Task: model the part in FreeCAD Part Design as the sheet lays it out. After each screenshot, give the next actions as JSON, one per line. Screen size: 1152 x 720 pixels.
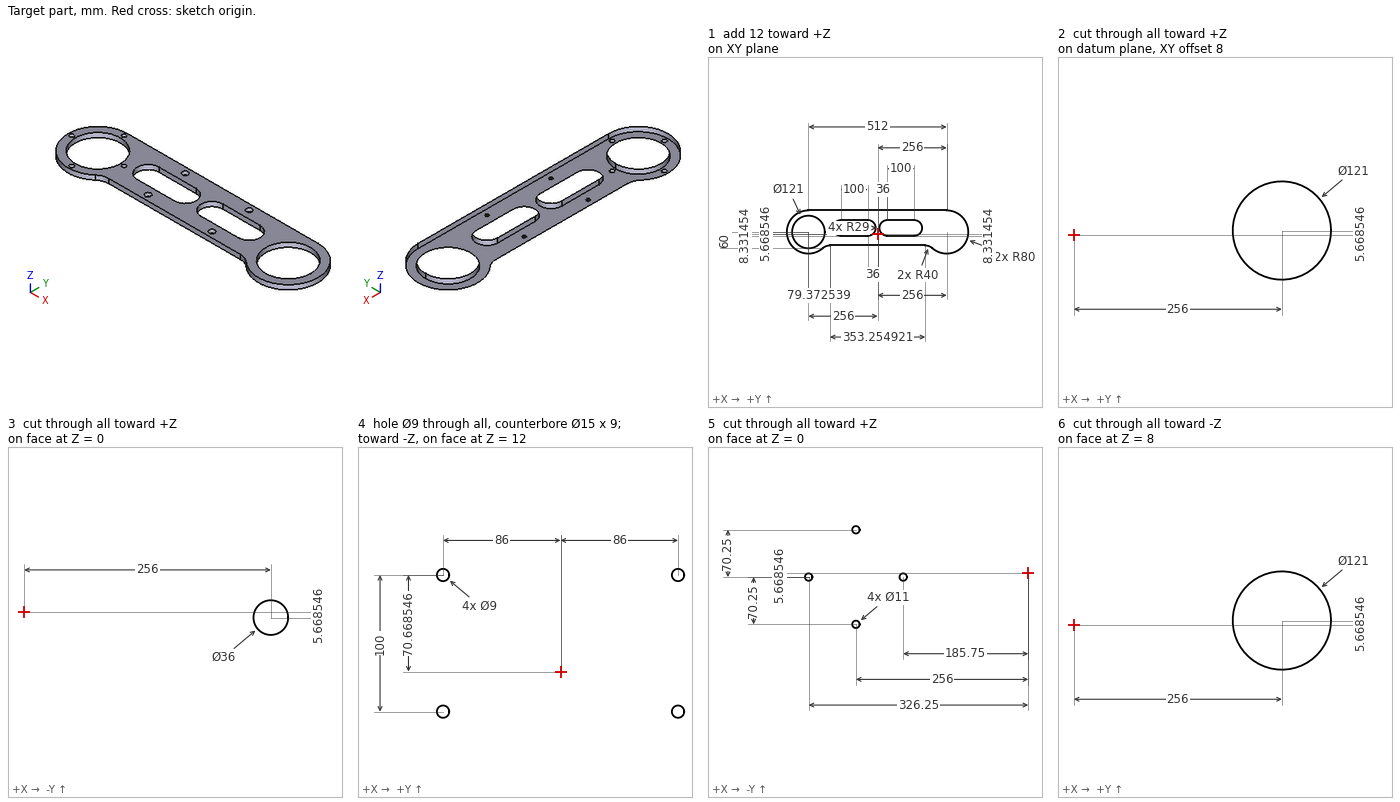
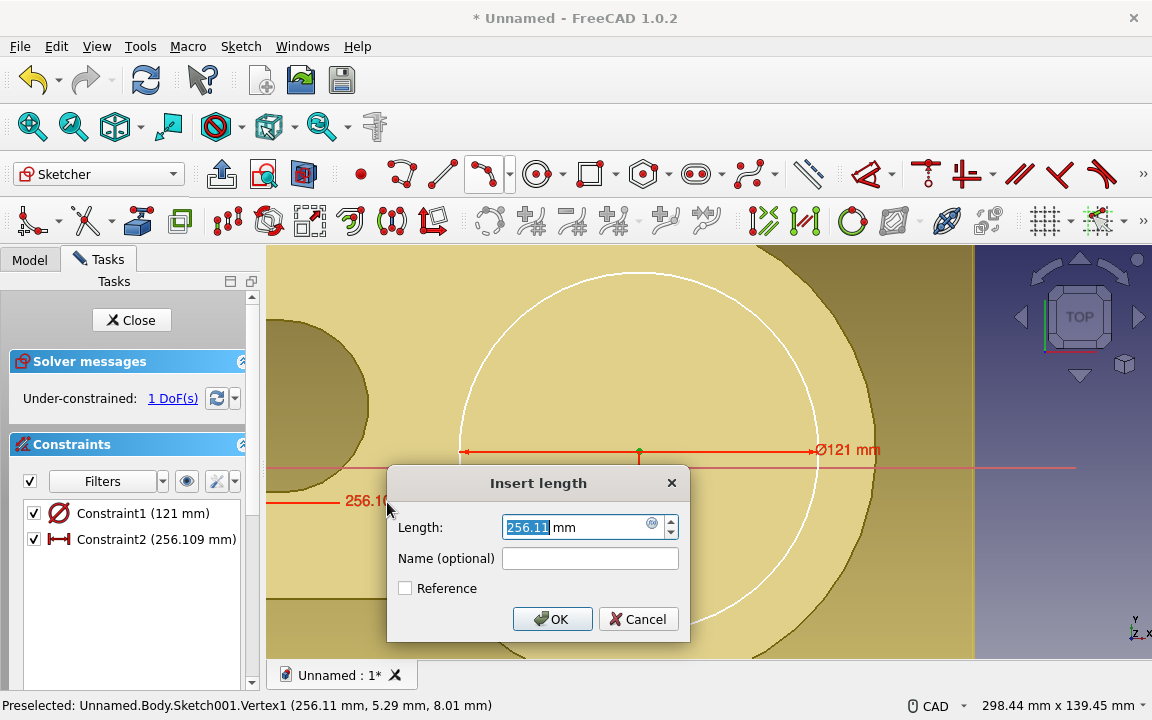
{"action": "type", "text": "256"}
{"action": "key", "text": "Return"}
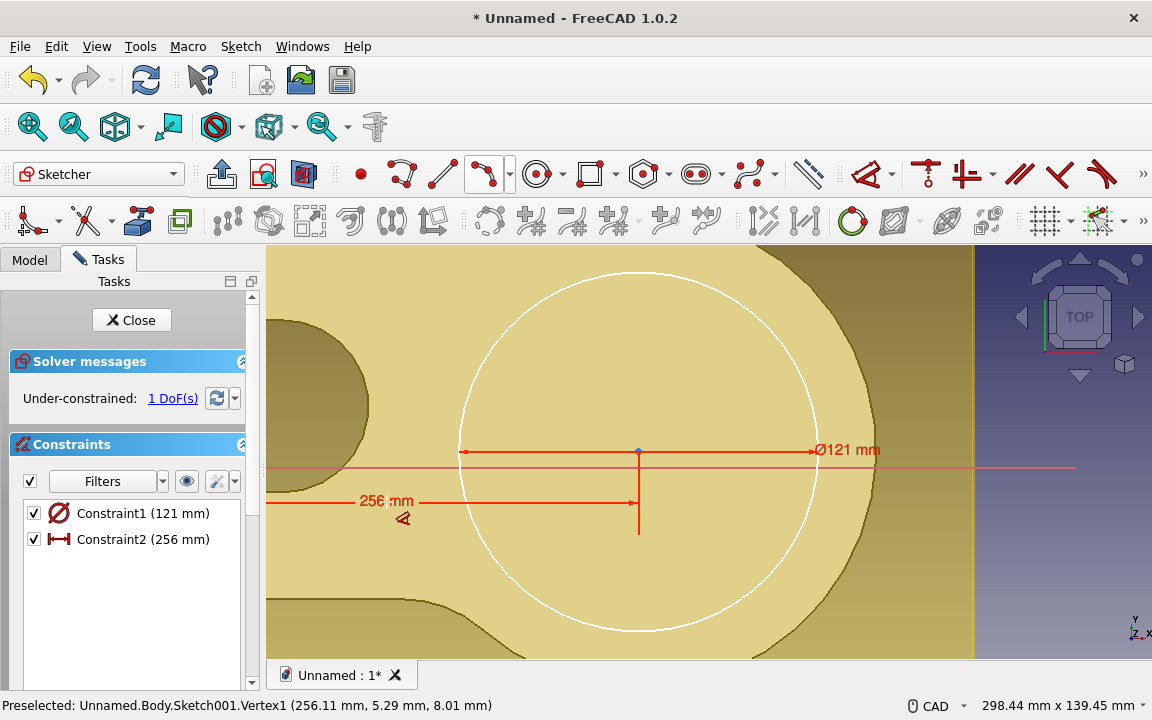
{"action": "scroll", "coordinate": [639, 452], "scroll_direction": "up", "scroll_amount": 5}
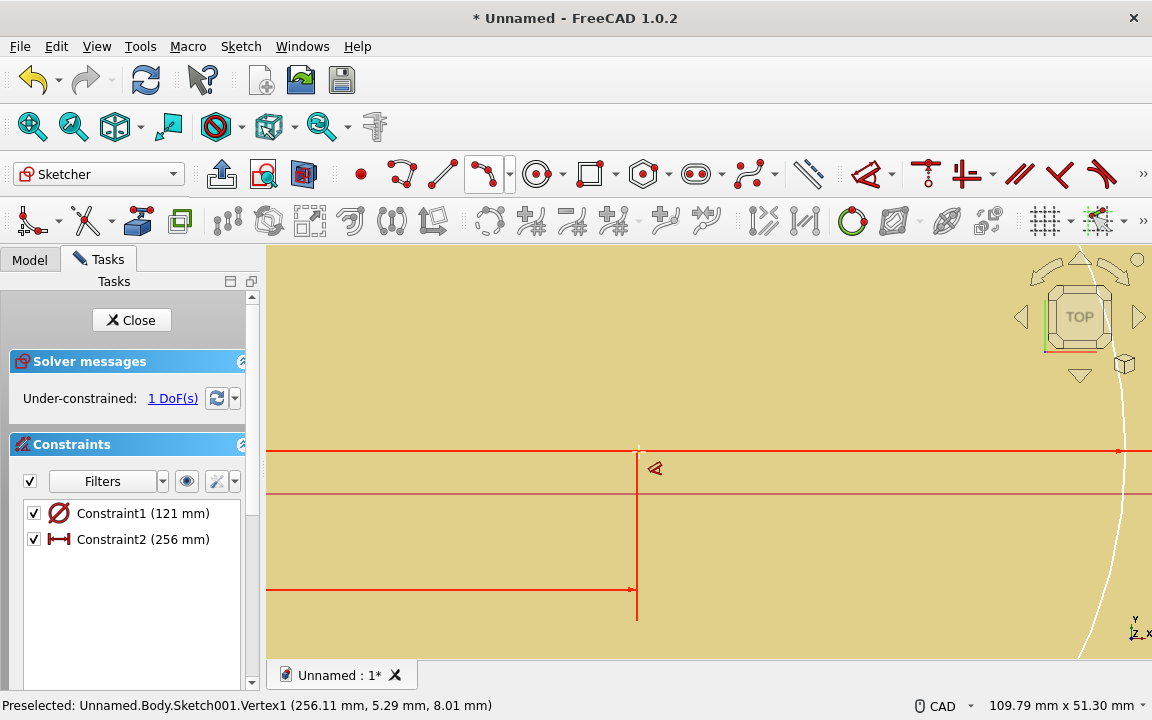
{"action": "left_click", "coordinate": [637, 451]}
{"action": "left_click", "coordinate": [671, 472]}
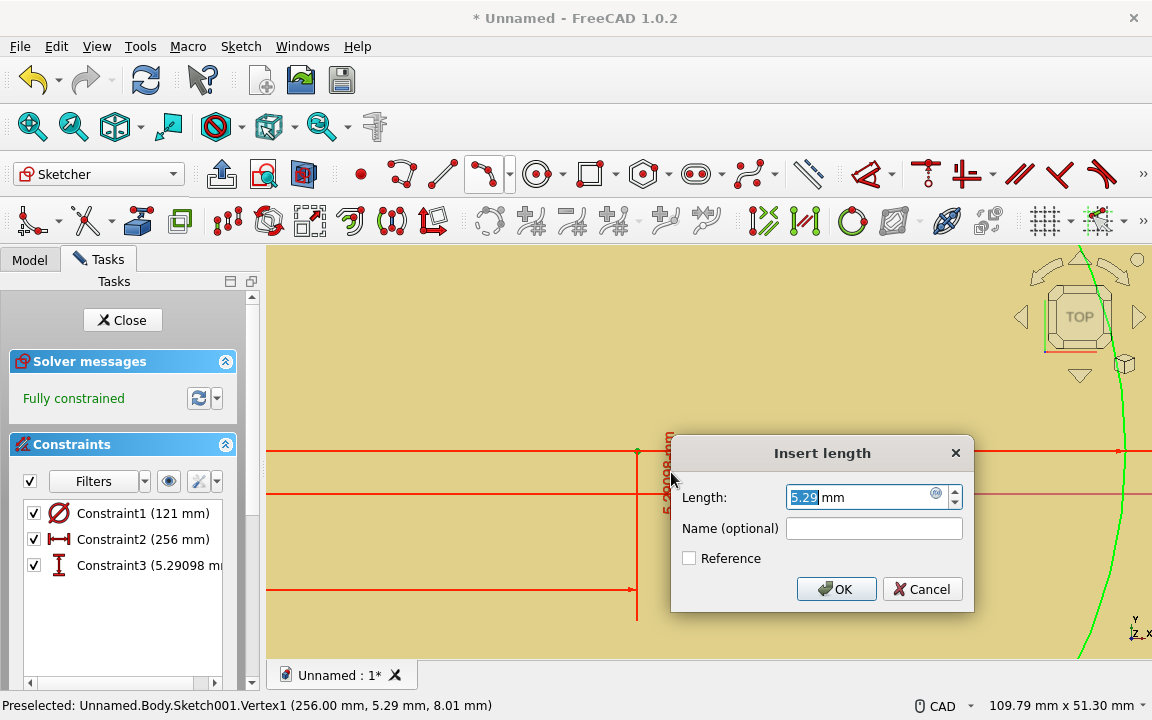
{"action": "type", "text": "5.668546"}
{"action": "key", "text": "Return"}
{"action": "key", "text": "Escape"}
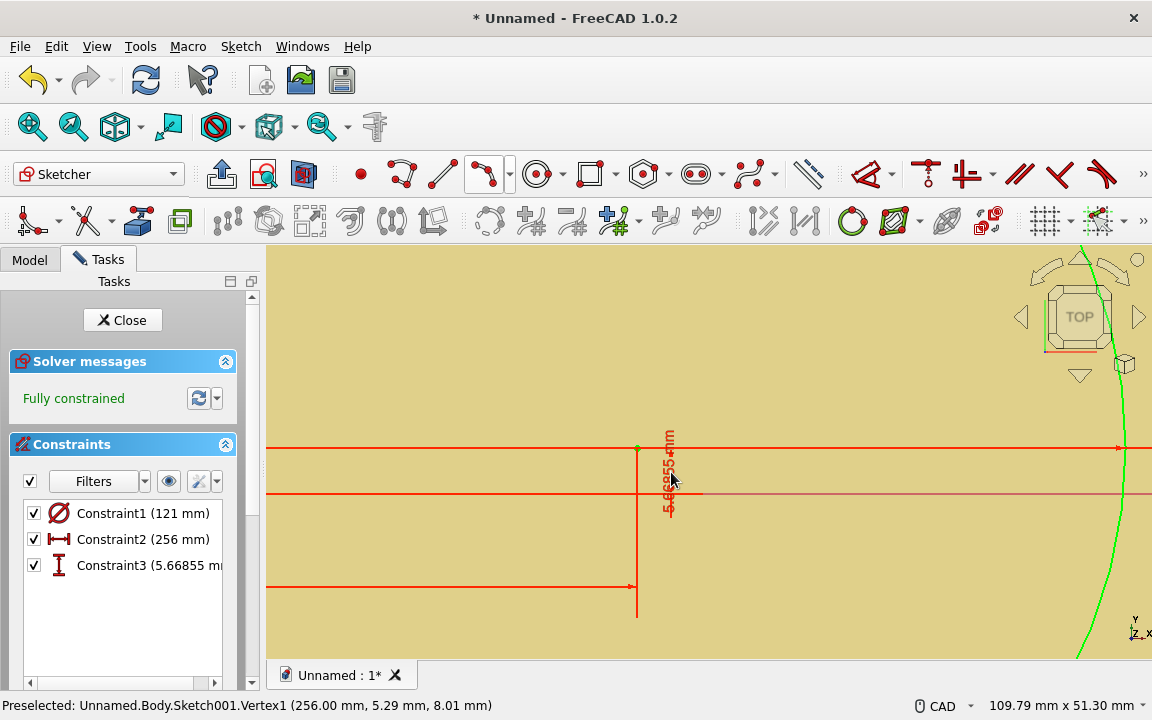
{"action": "left_click", "coordinate": [123, 320]}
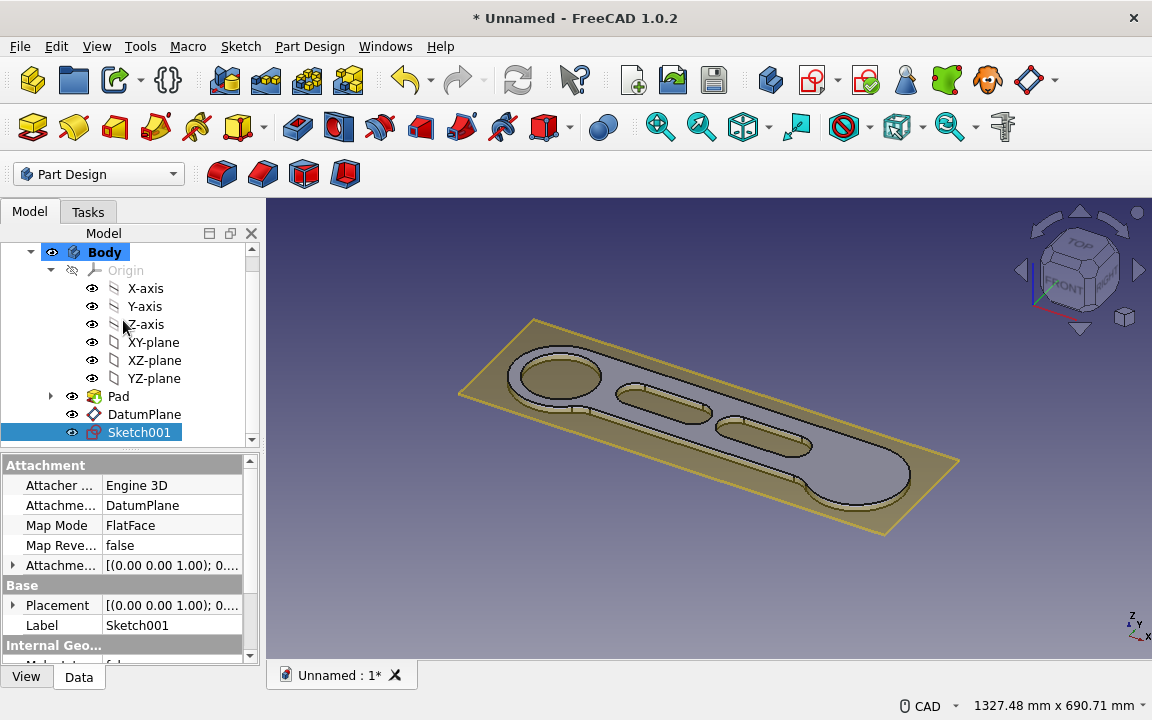
{"action": "left_click", "coordinate": [298, 128]}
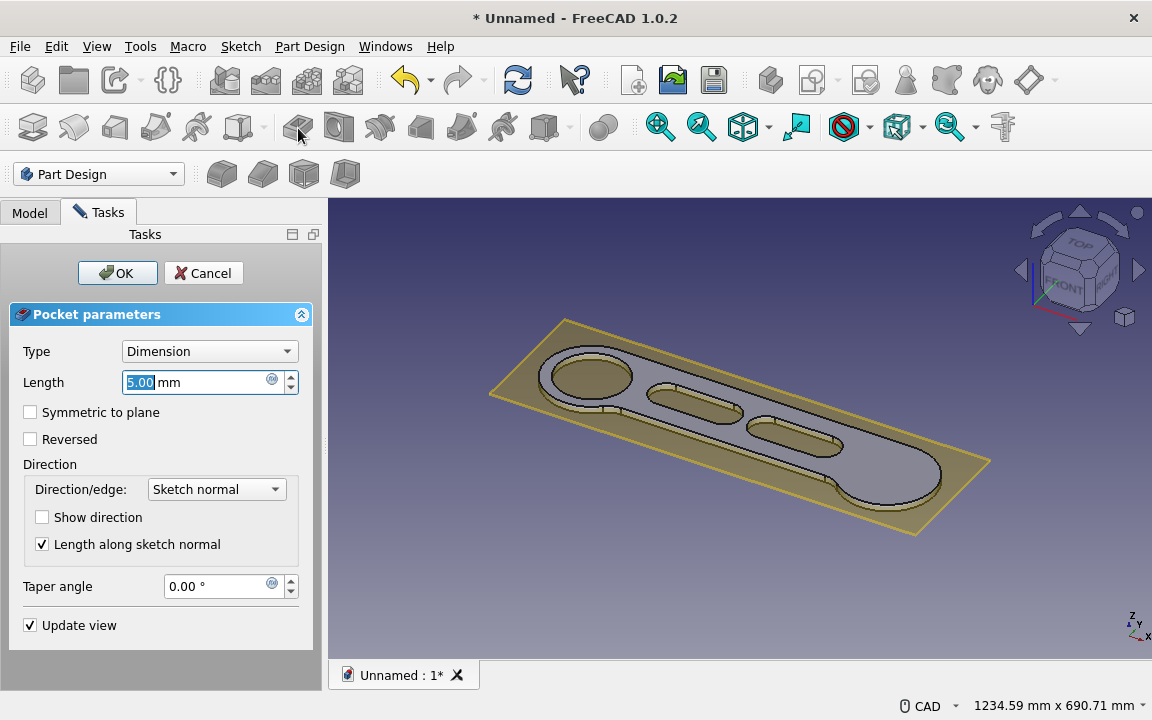
{"action": "left_click", "coordinate": [210, 352]}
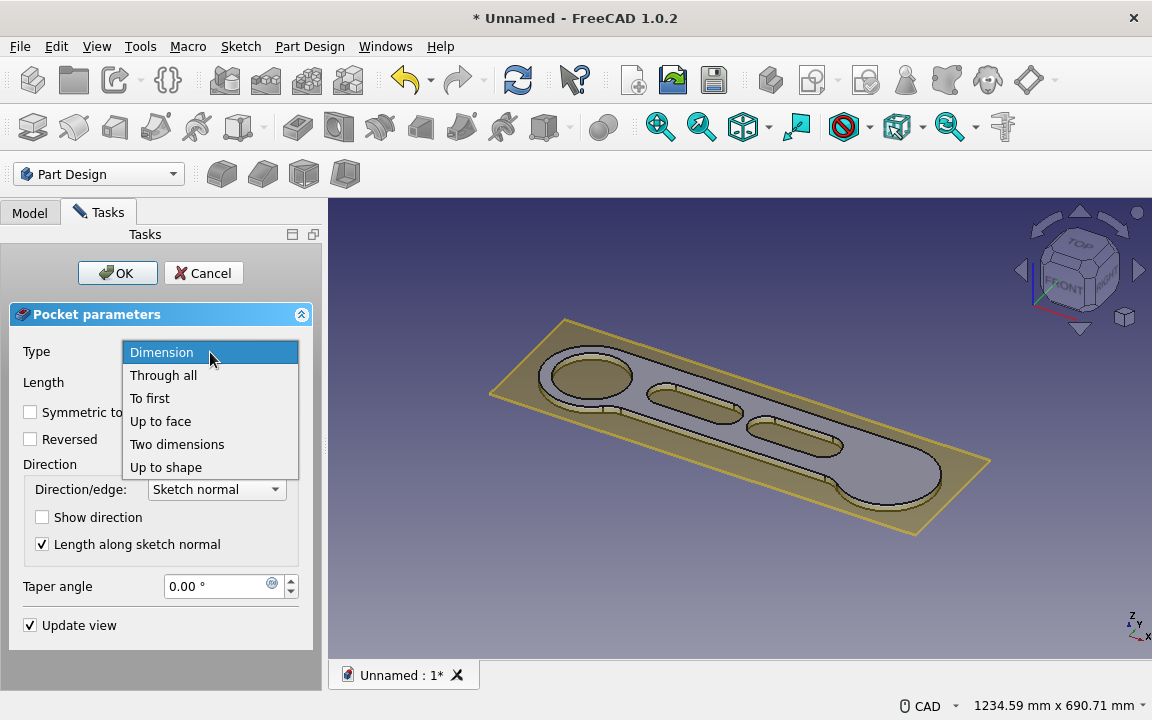
{"action": "left_click", "coordinate": [208, 376]}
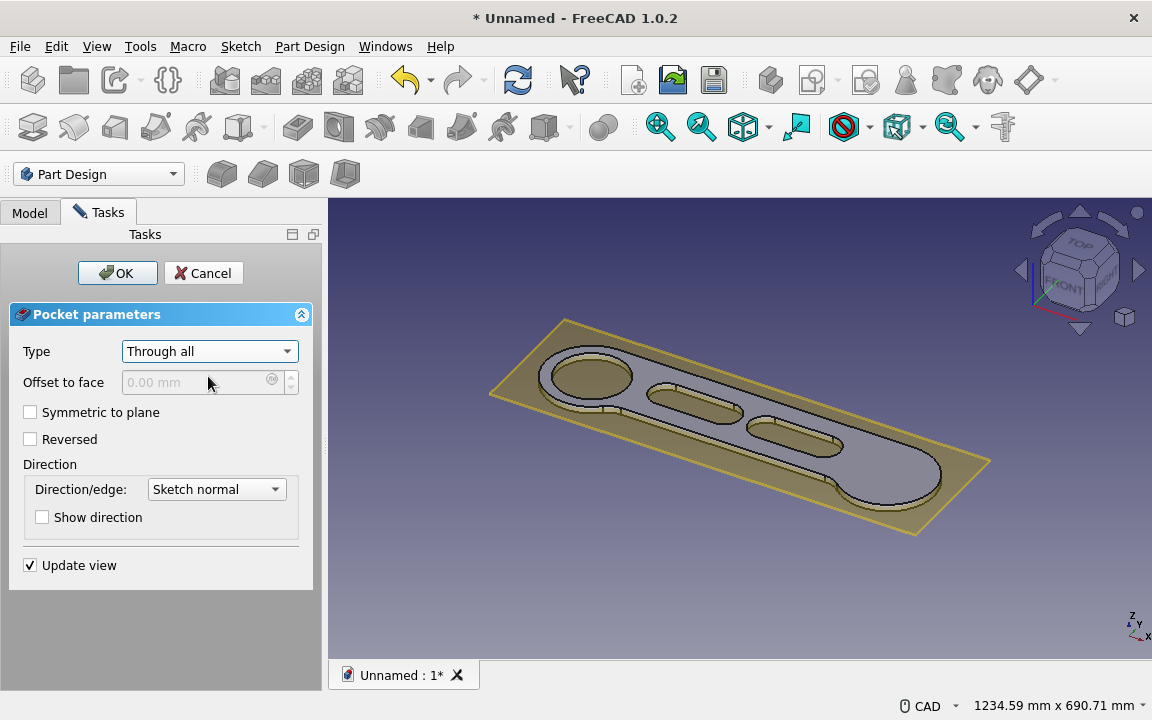
{"action": "left_click", "coordinate": [31, 439]}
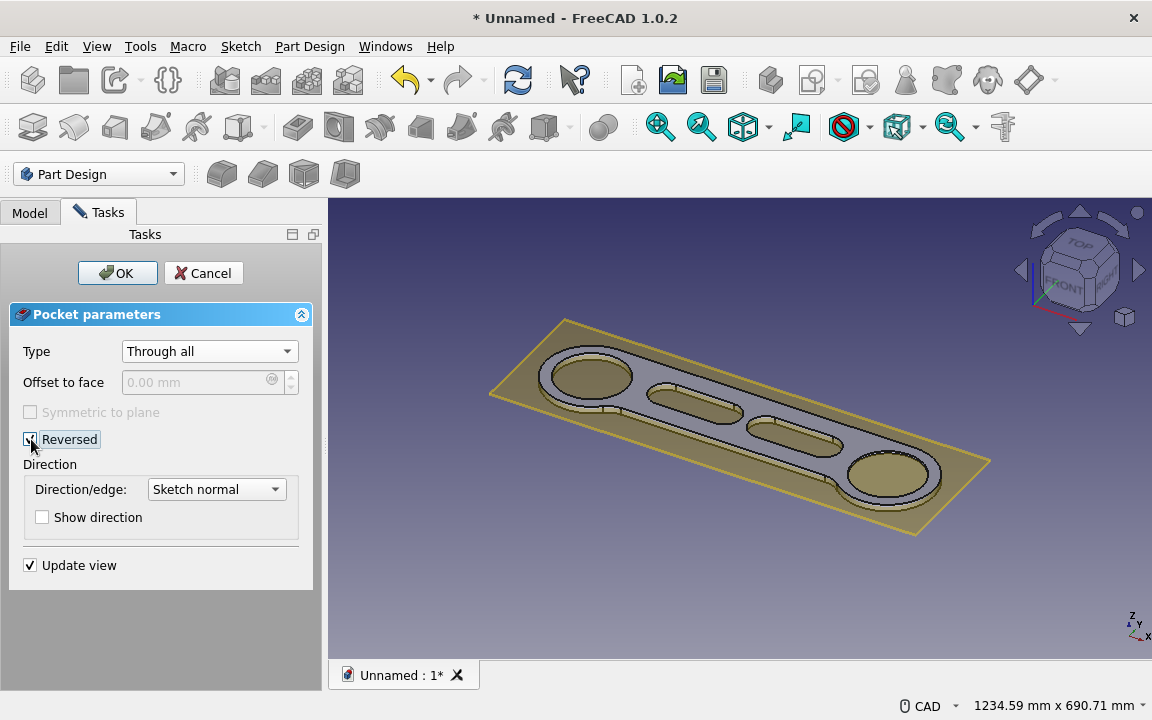
{"action": "left_click", "coordinate": [118, 273]}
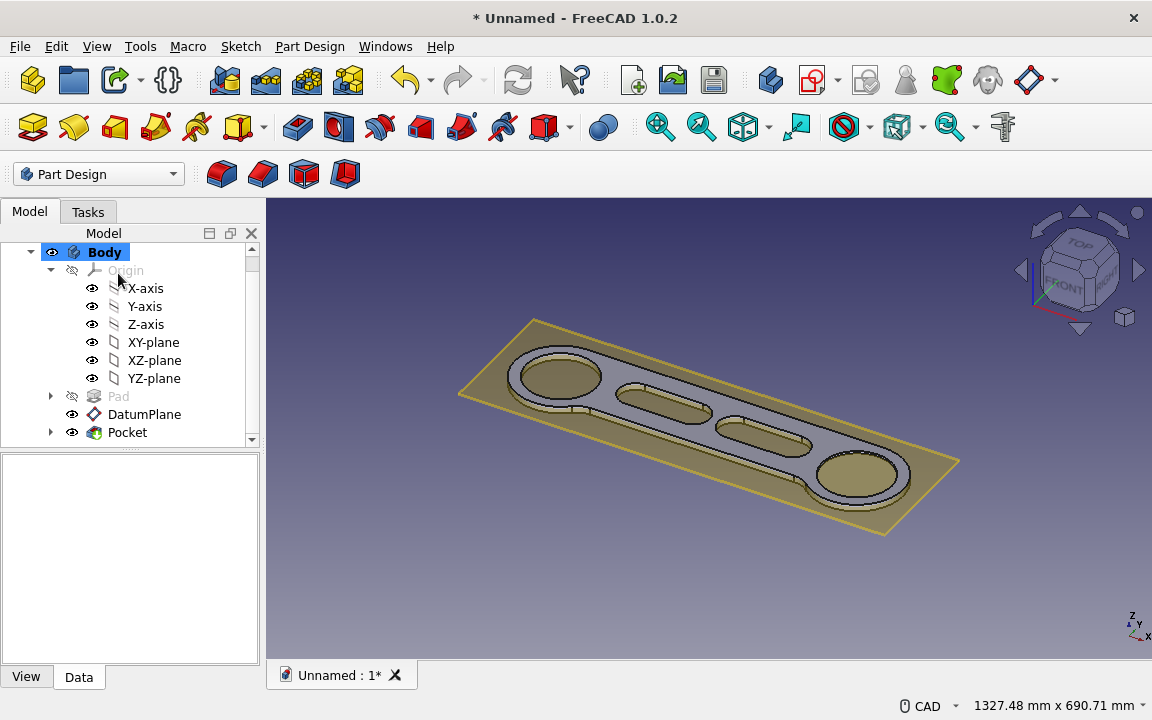
{"action": "left_click", "coordinate": [117, 414]}
{"action": "key", "text": "space"}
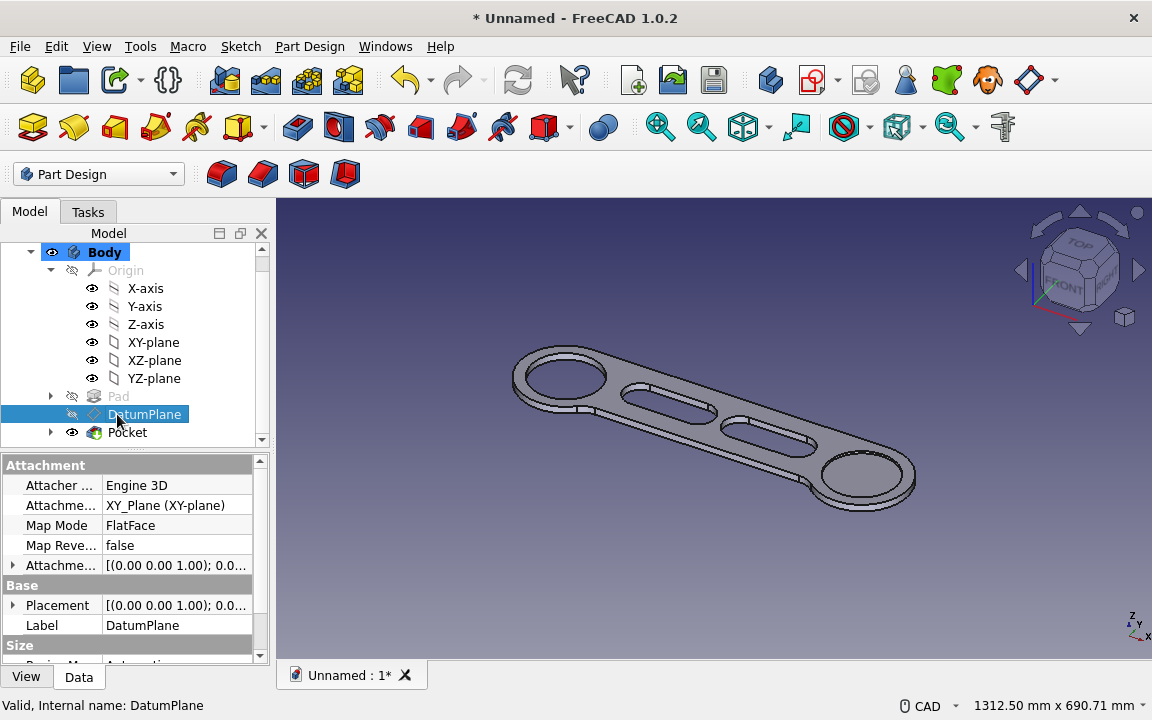
{"action": "key", "text": "5"}